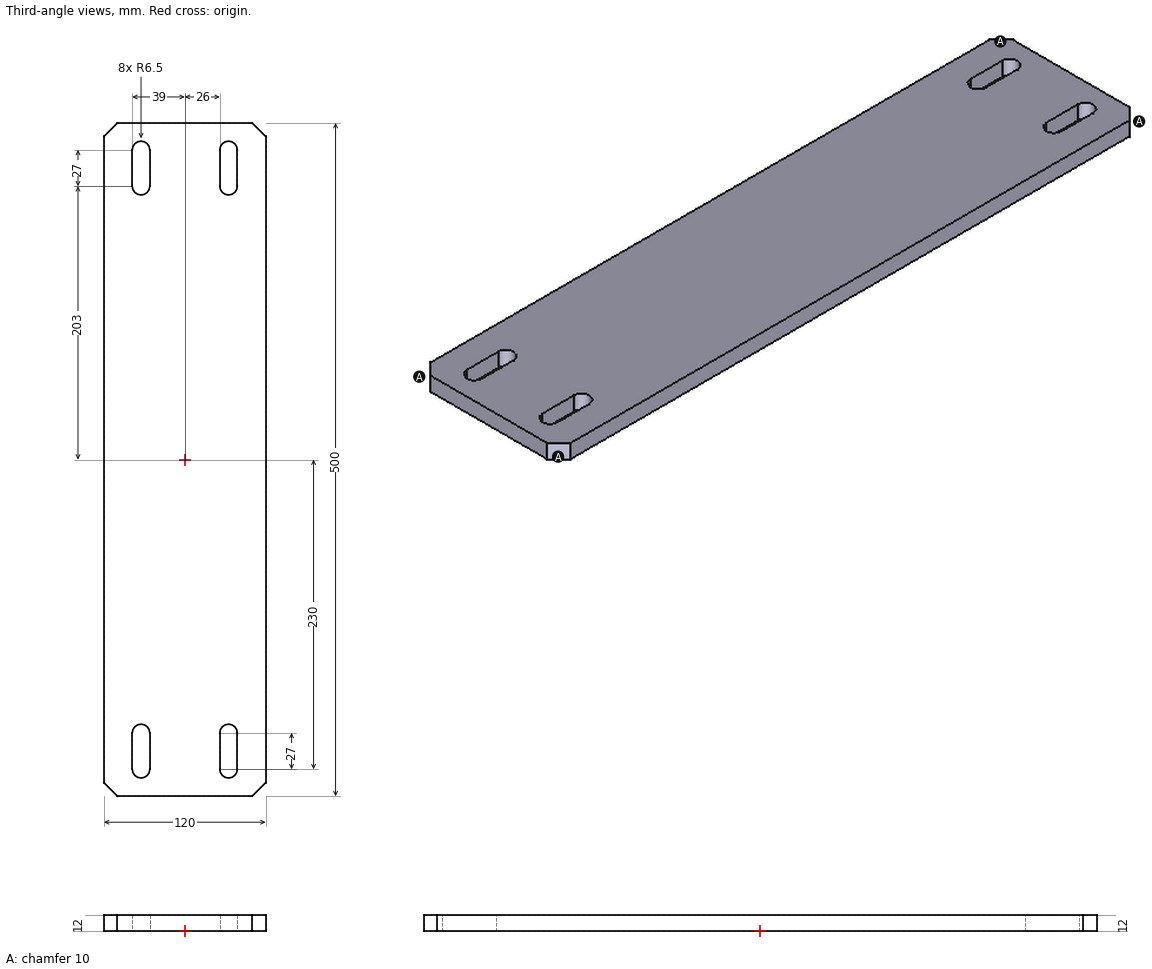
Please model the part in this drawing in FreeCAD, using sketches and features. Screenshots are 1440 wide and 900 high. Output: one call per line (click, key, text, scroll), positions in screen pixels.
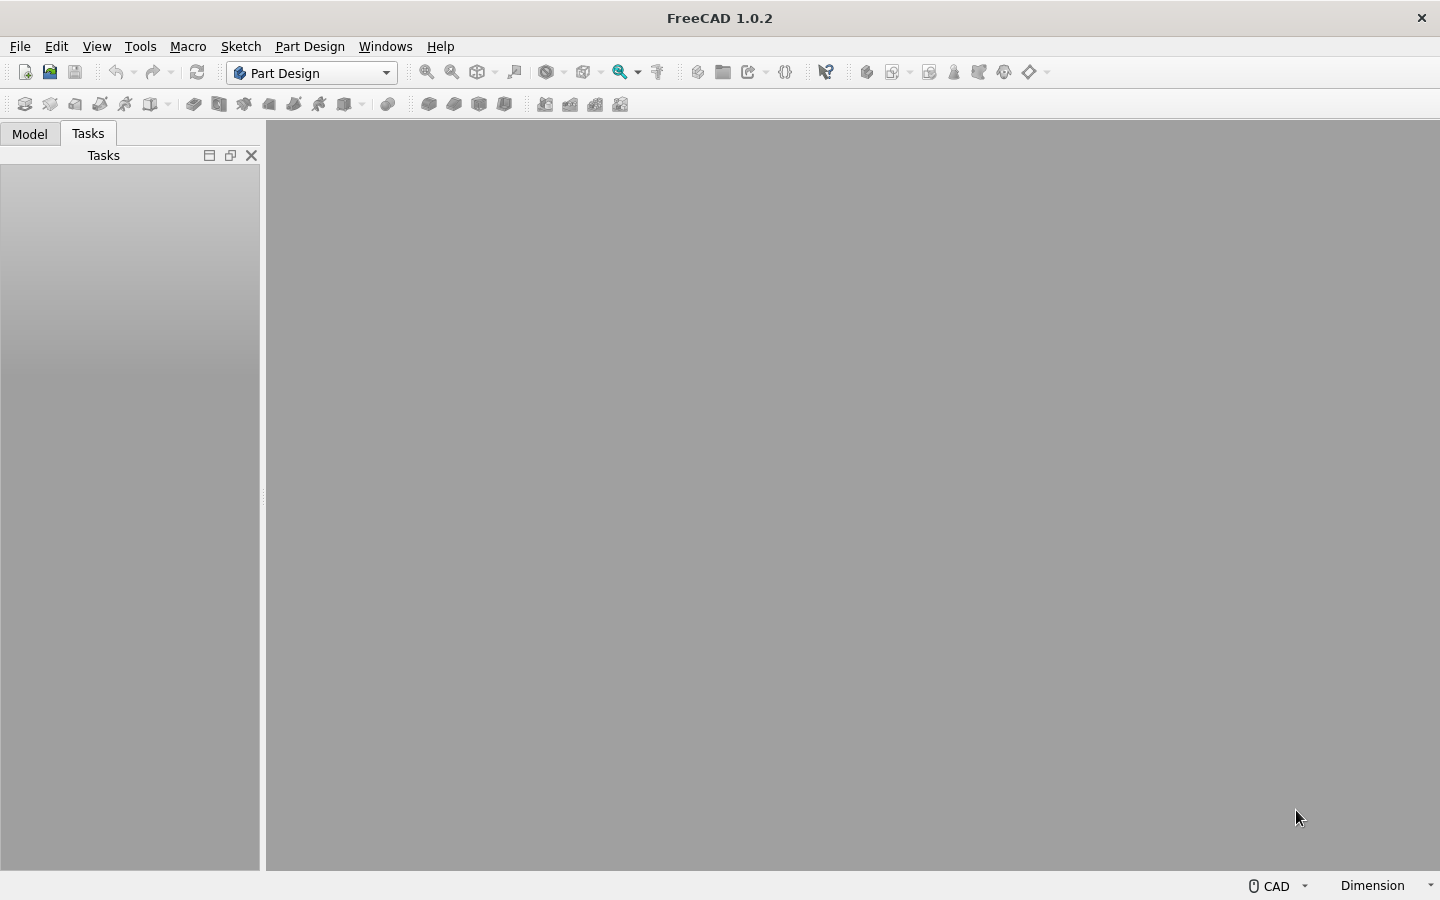
key(ctrl+n)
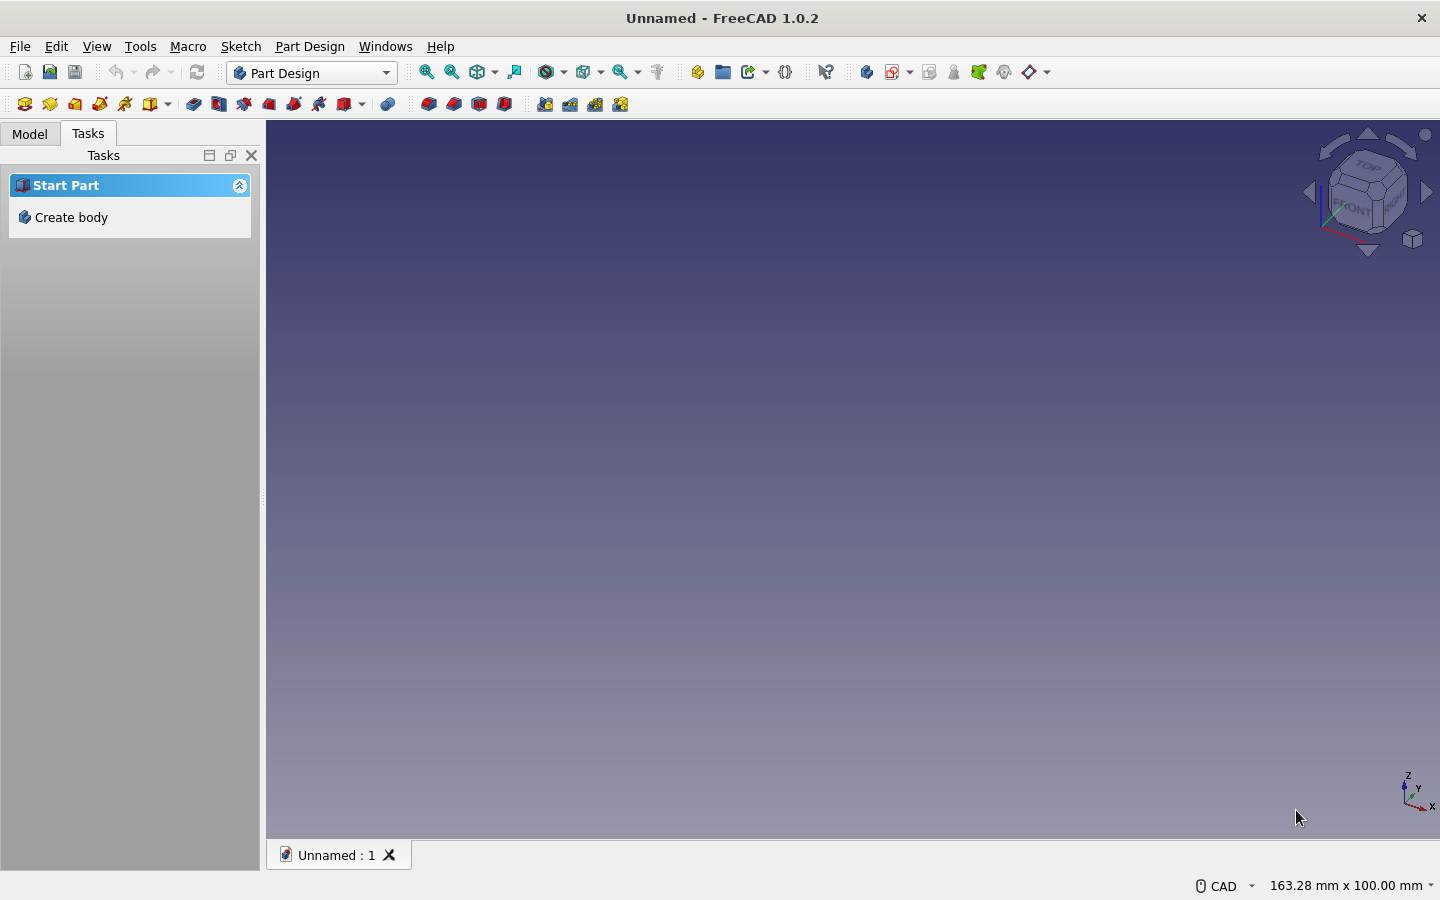
click(892, 72)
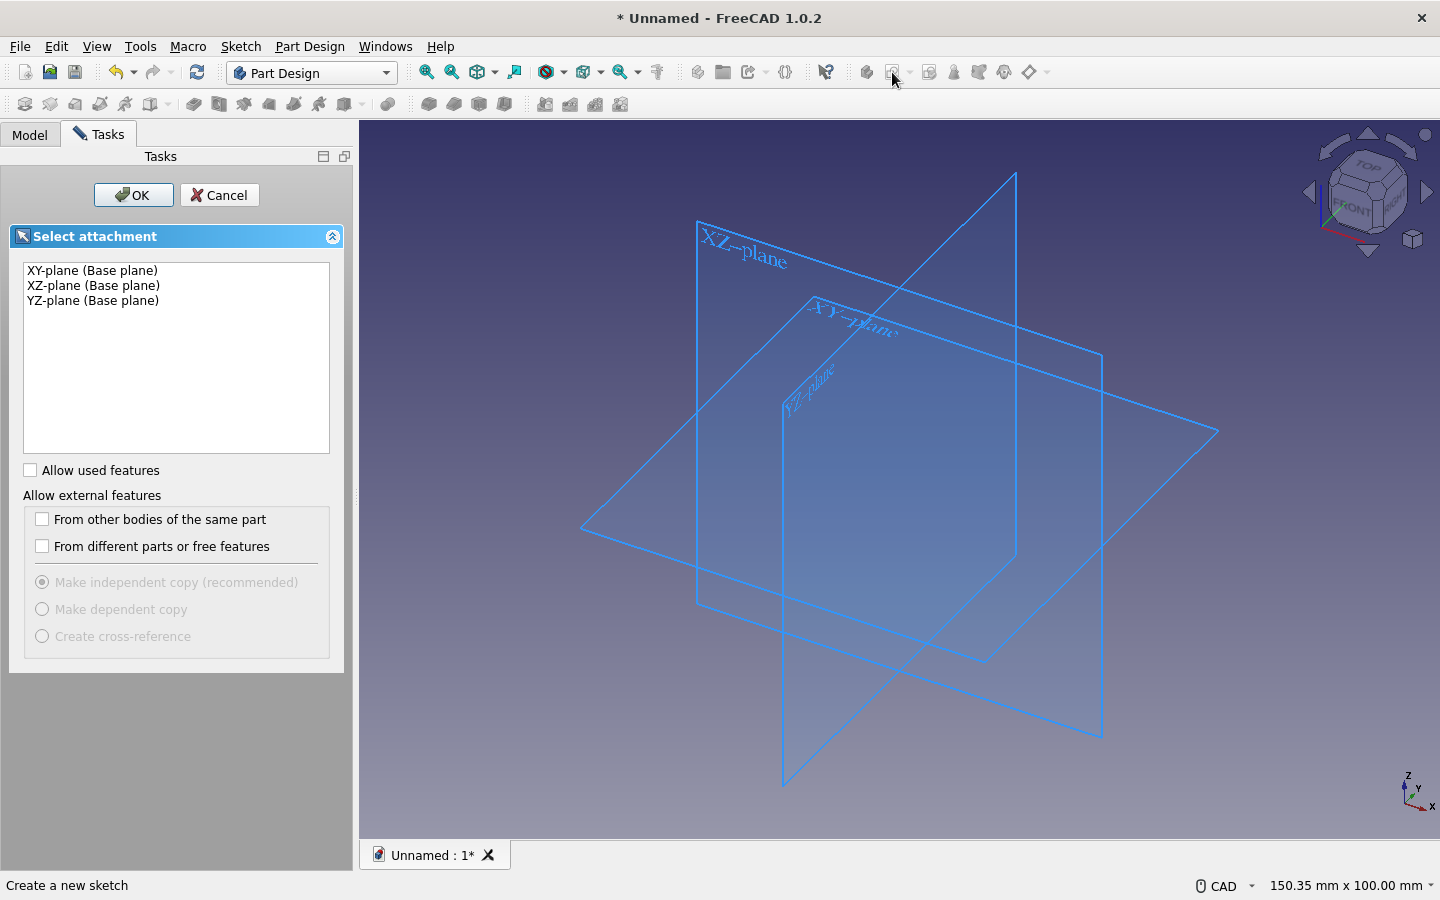
click(84, 270)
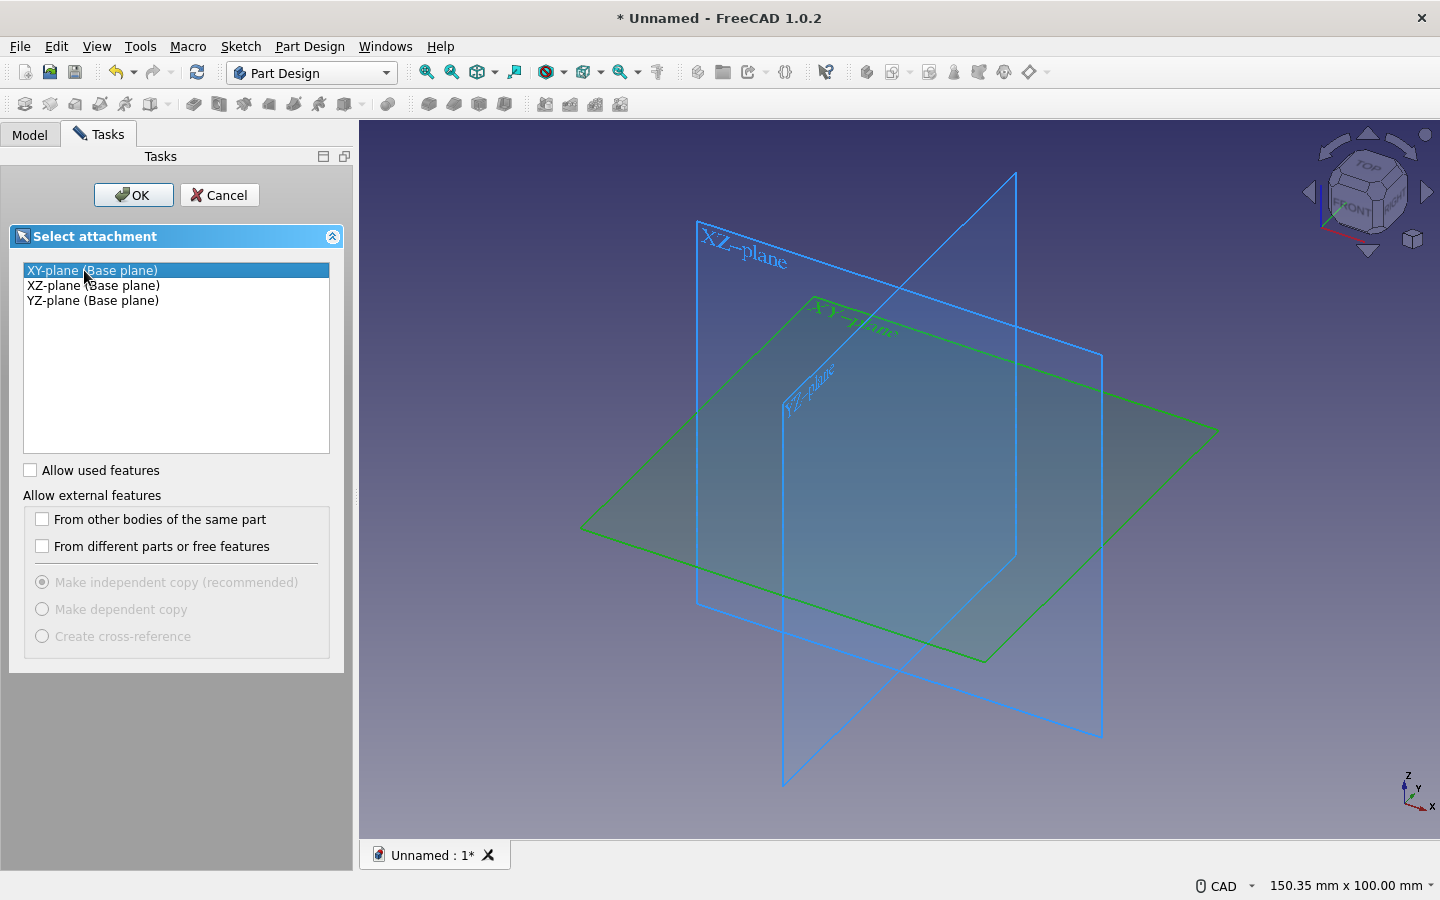
click(134, 195)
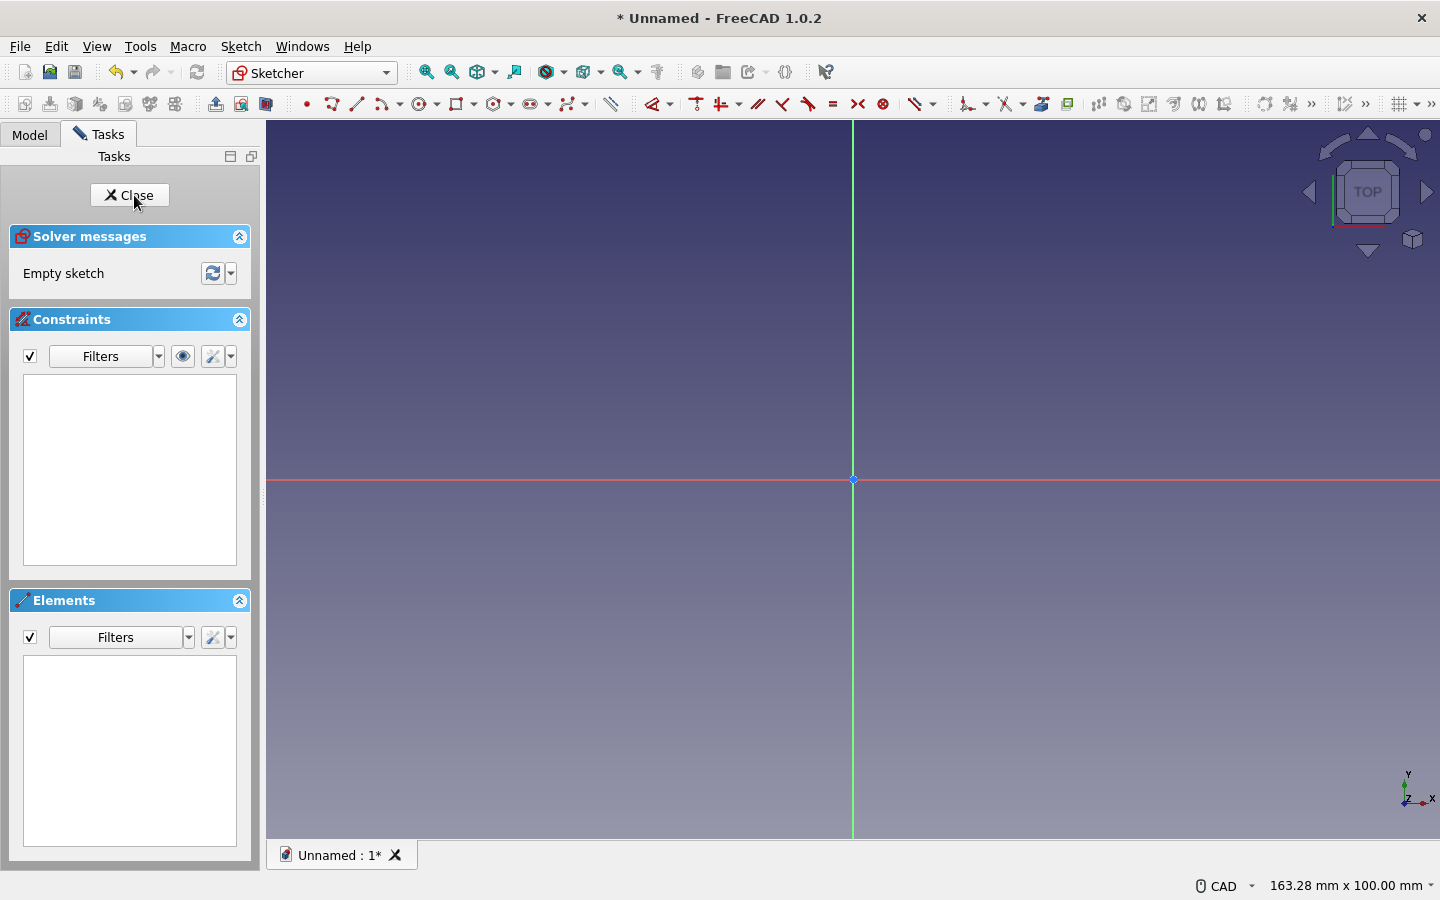
scroll(774, 480, down, 10)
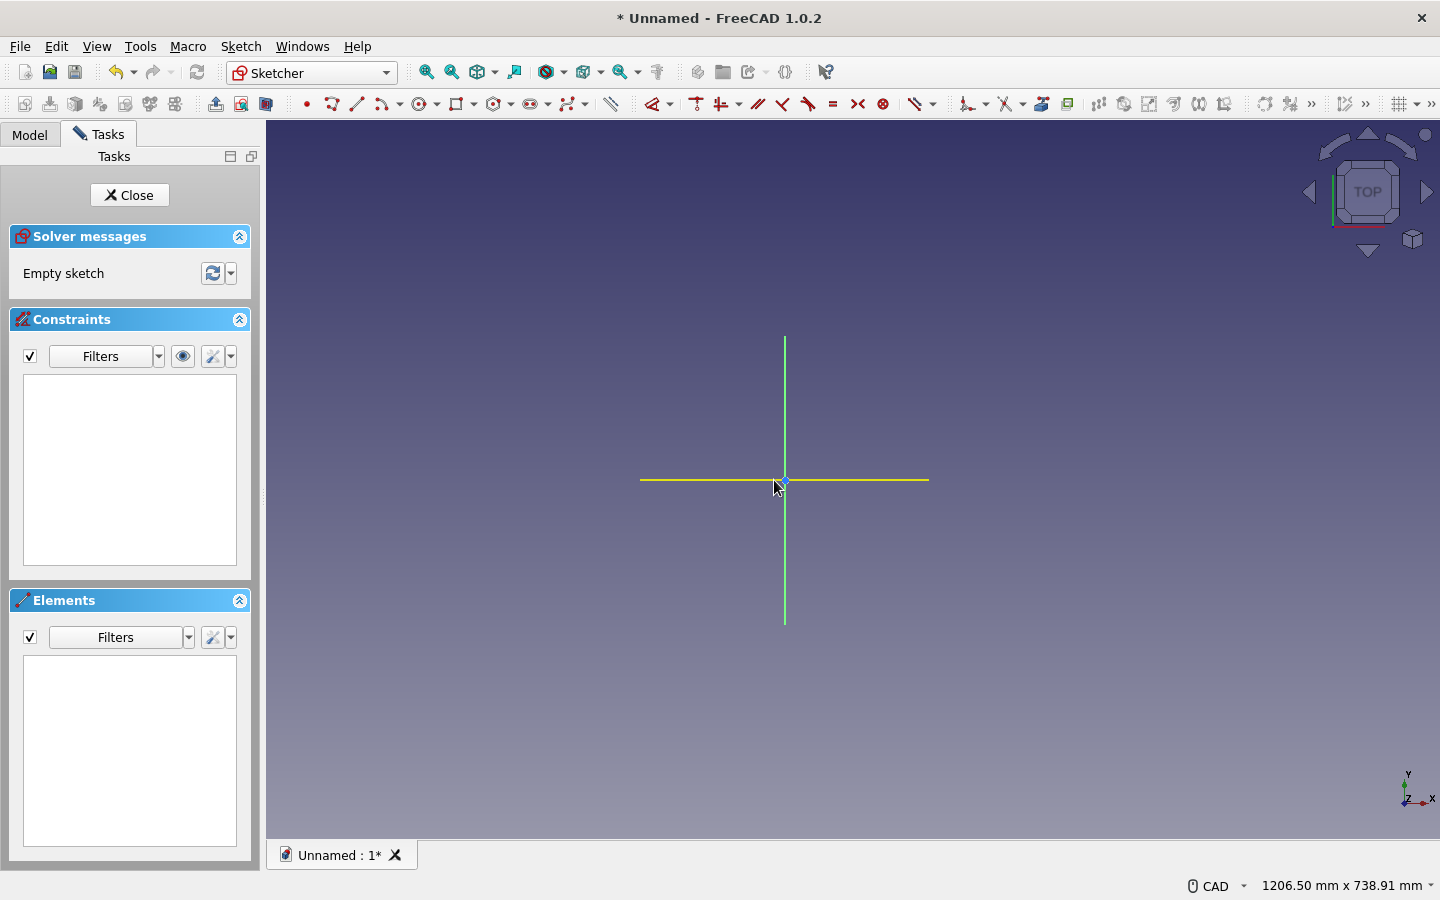
key(g)
key(v)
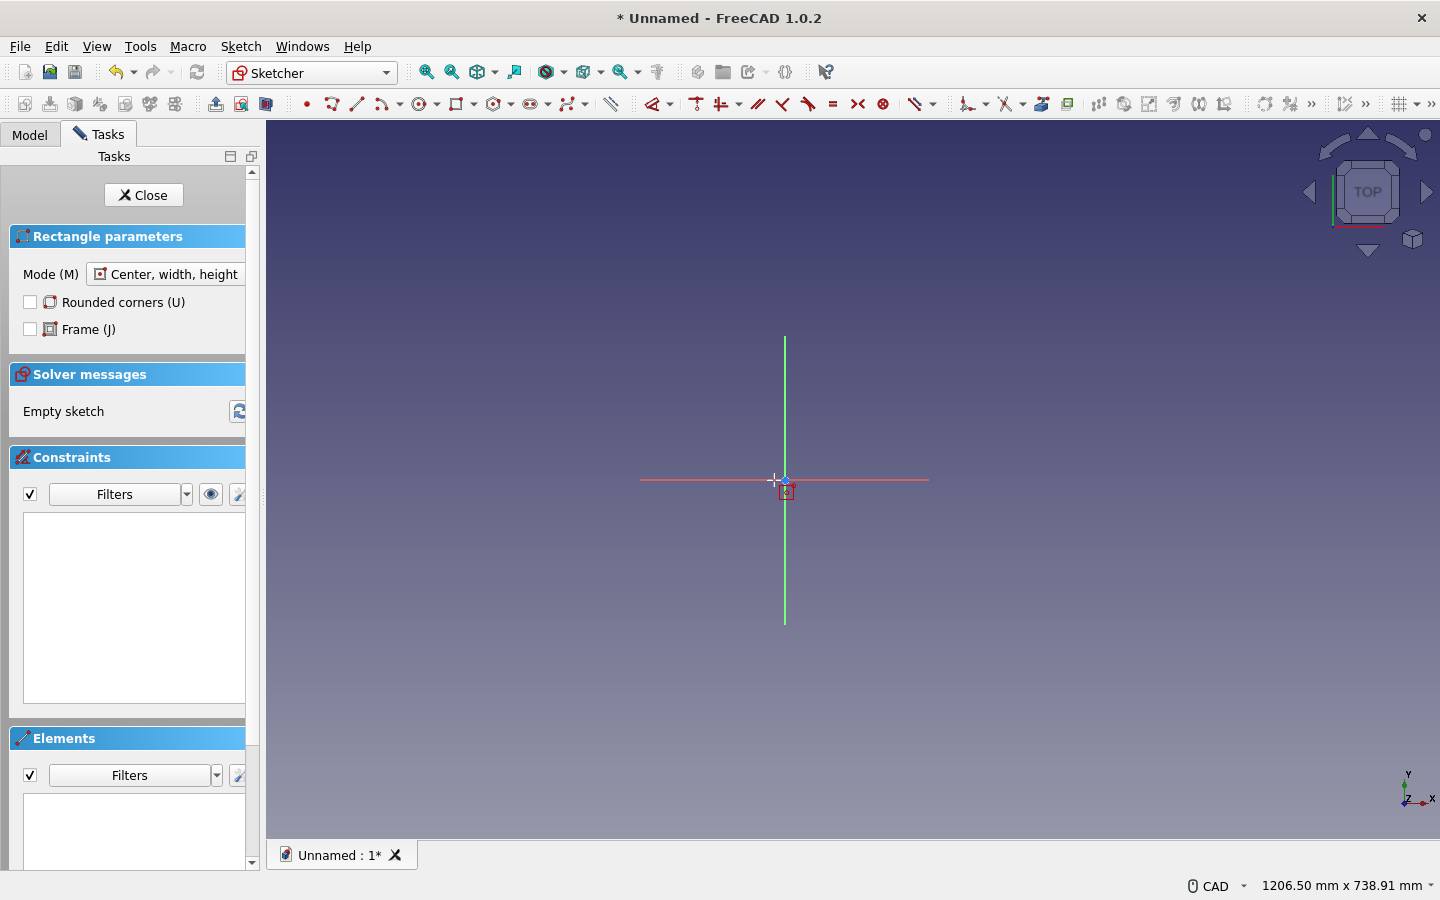
click(785, 480)
move(843, 237)